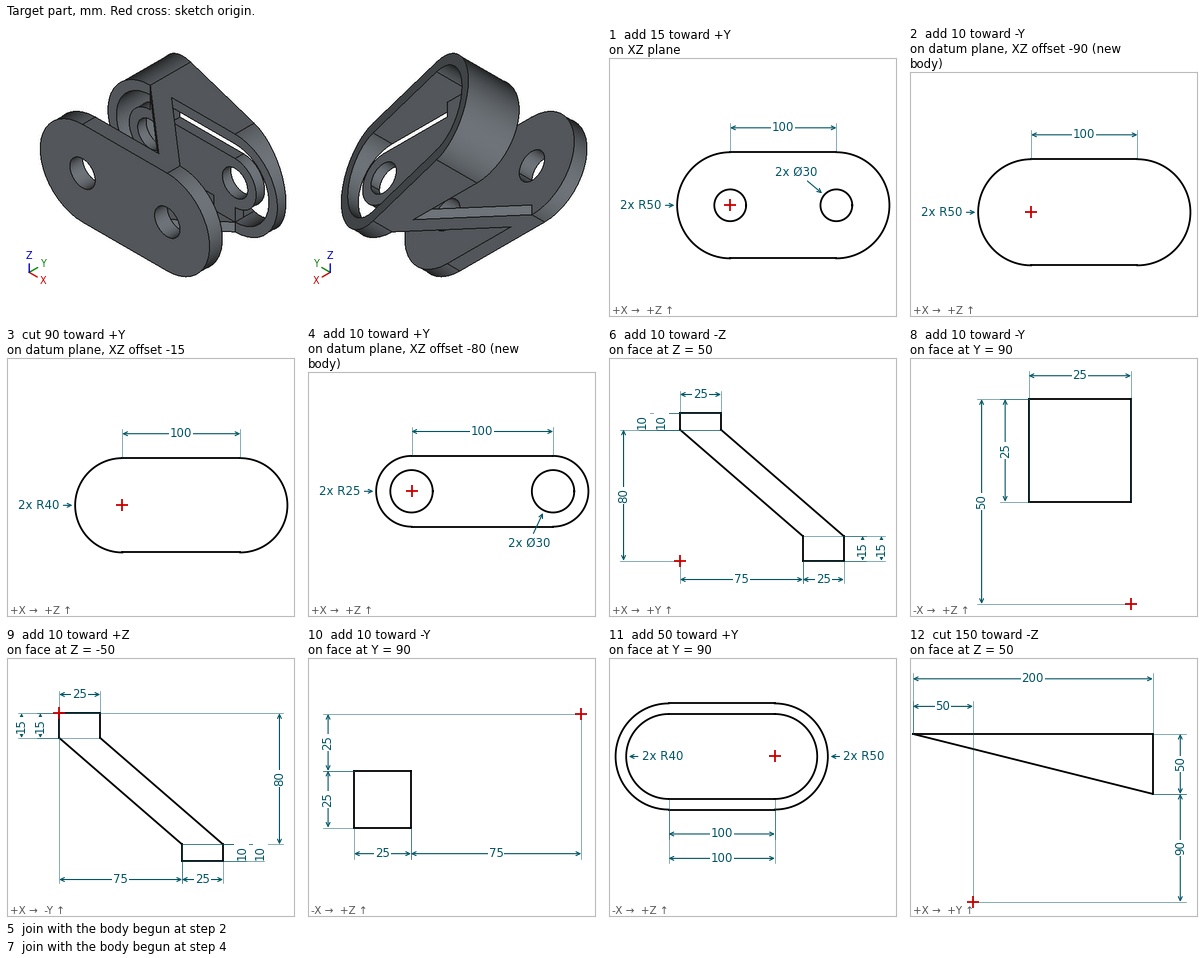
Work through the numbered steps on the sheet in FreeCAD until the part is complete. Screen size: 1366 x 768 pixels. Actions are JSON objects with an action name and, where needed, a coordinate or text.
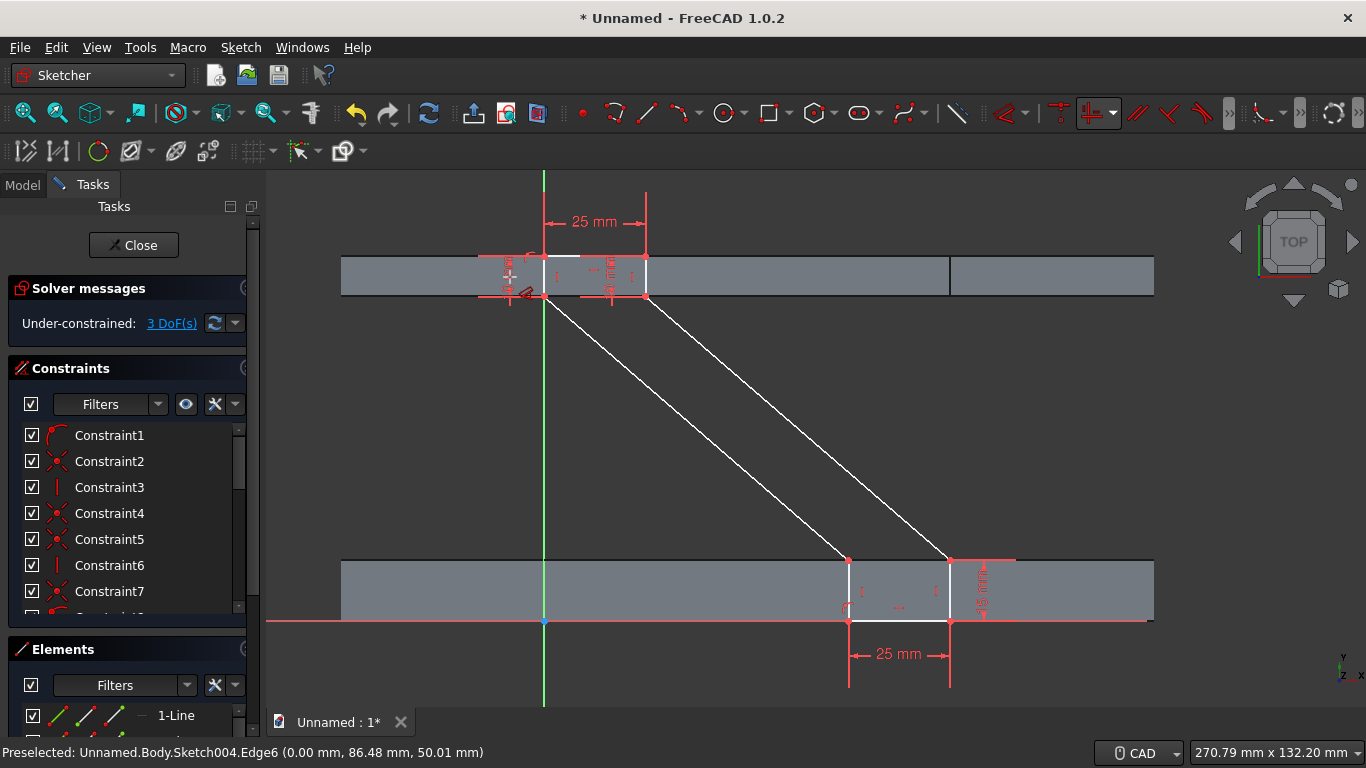
{"action": "left_click", "coordinate": [849, 579]}
{"action": "left_click", "coordinate": [883, 591]}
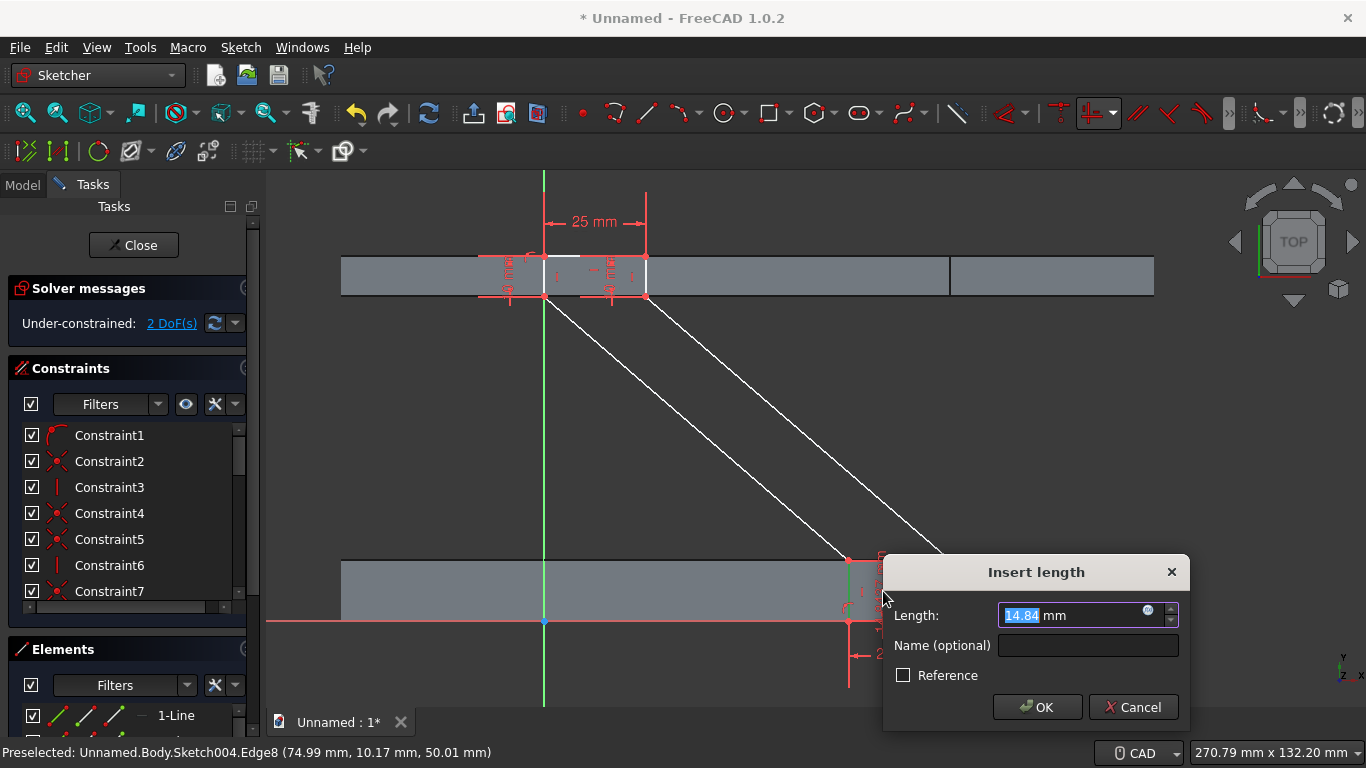
{"action": "type", "text": "15"}
{"action": "key", "text": "Return"}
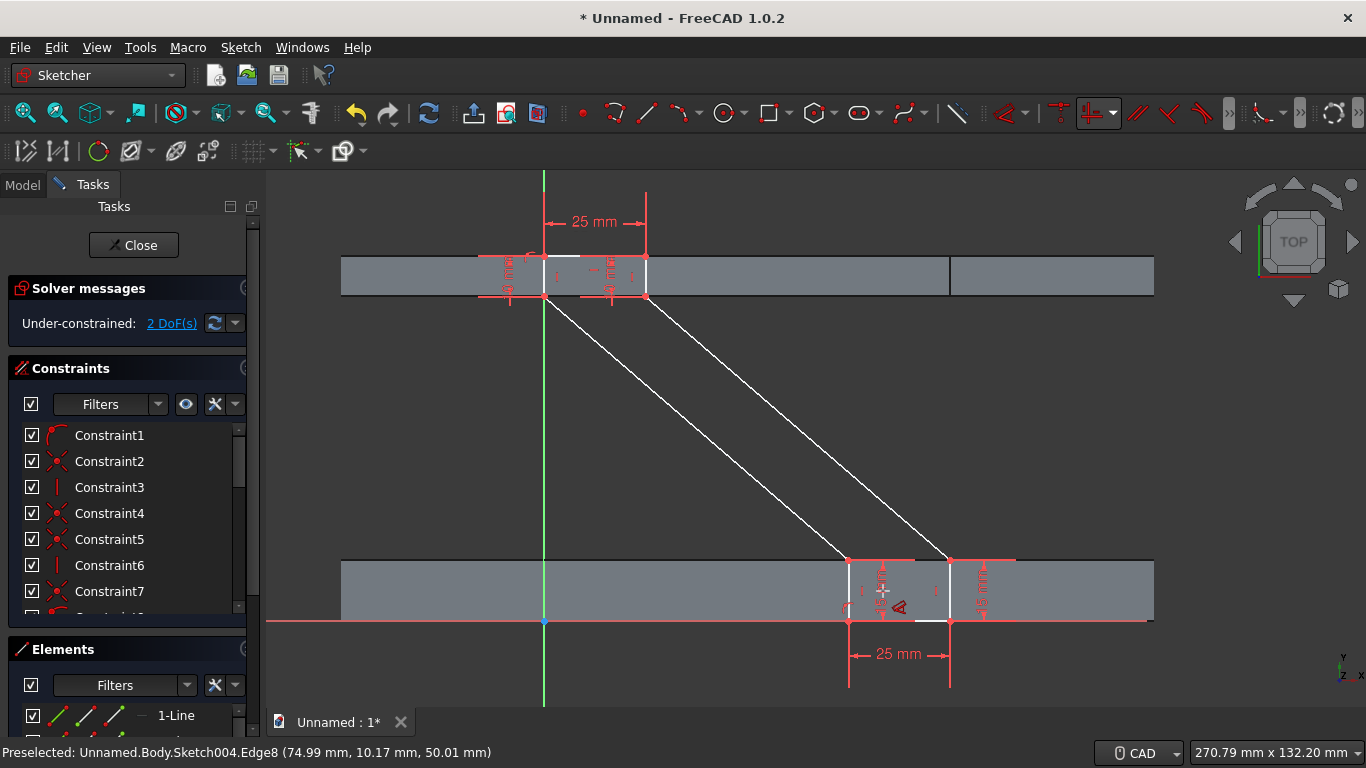
{"action": "left_click", "coordinate": [849, 621]}
{"action": "left_click", "coordinate": [696, 655]}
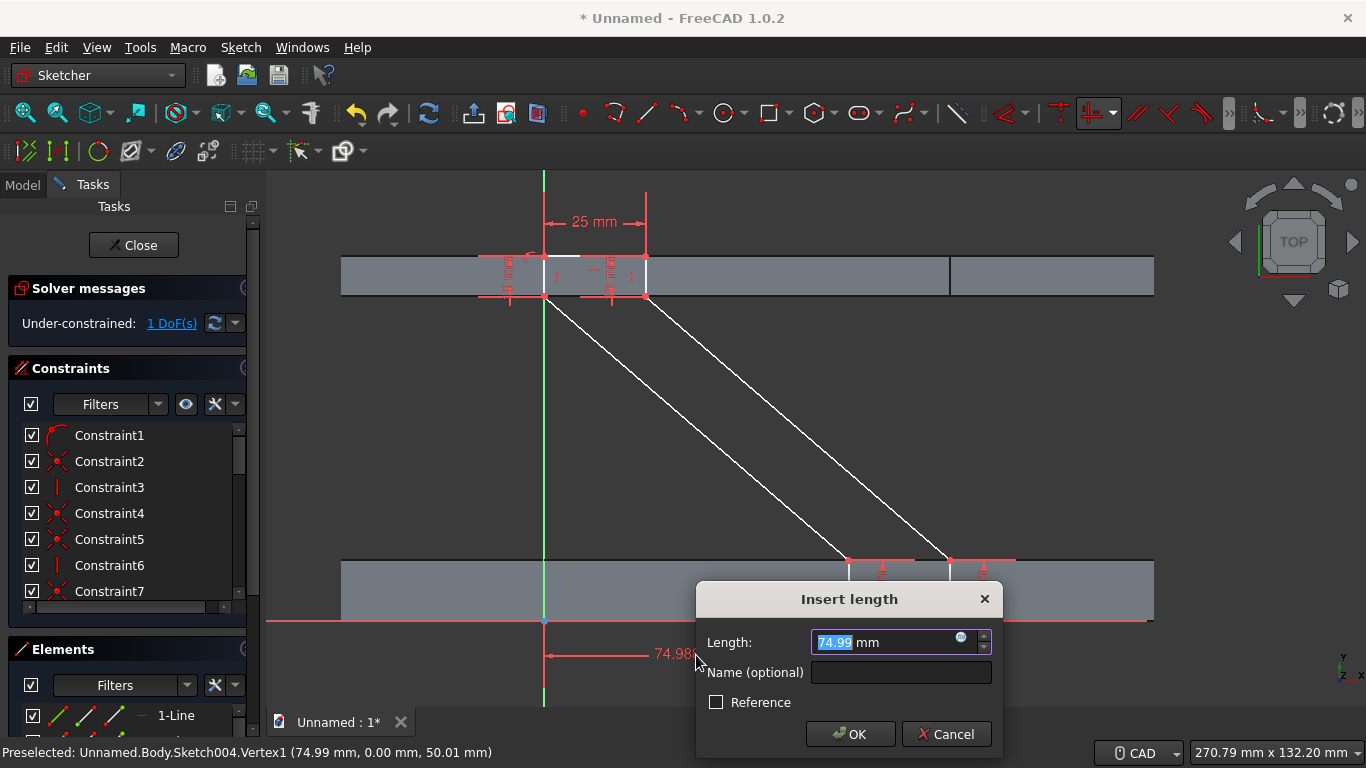
{"action": "type", "text": "75"}
{"action": "key", "text": "Return"}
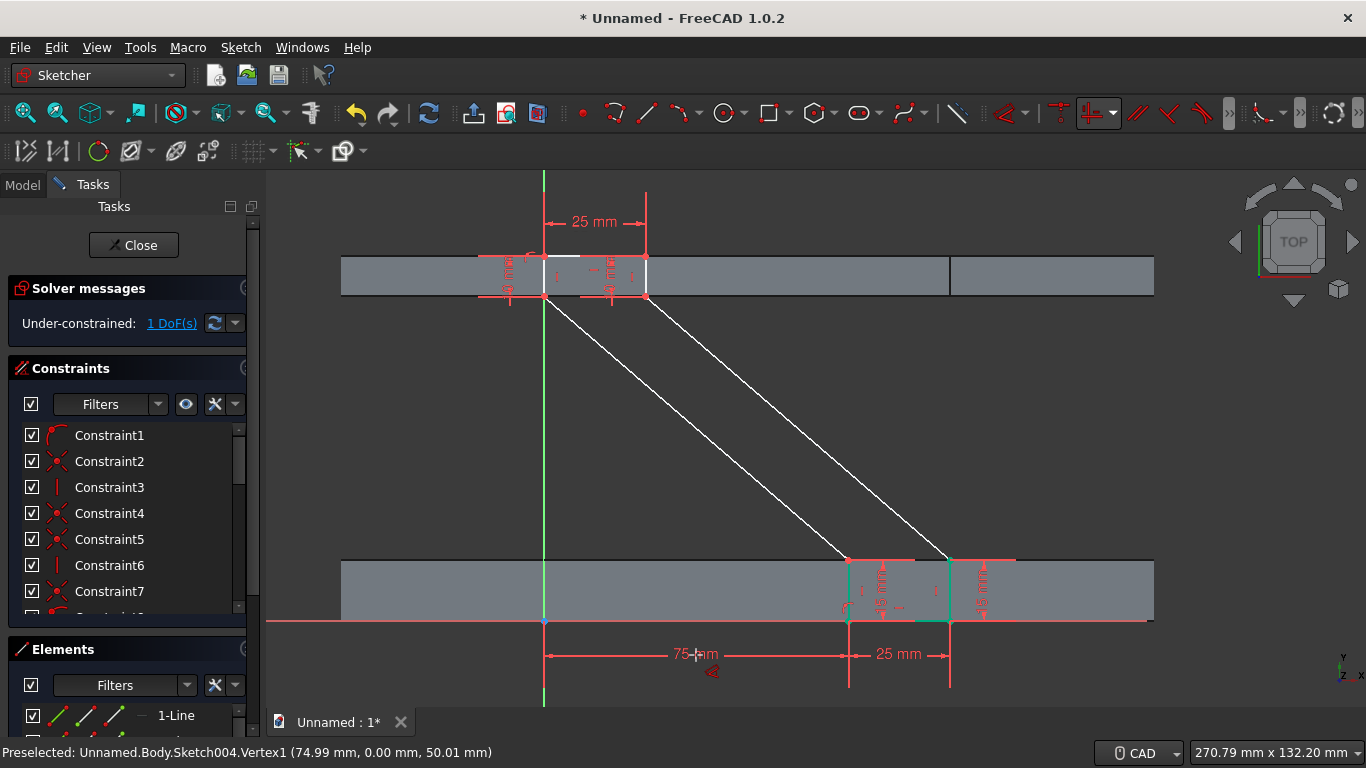
{"action": "left_click", "coordinate": [646, 297]}
{"action": "left_click", "coordinate": [510, 459]}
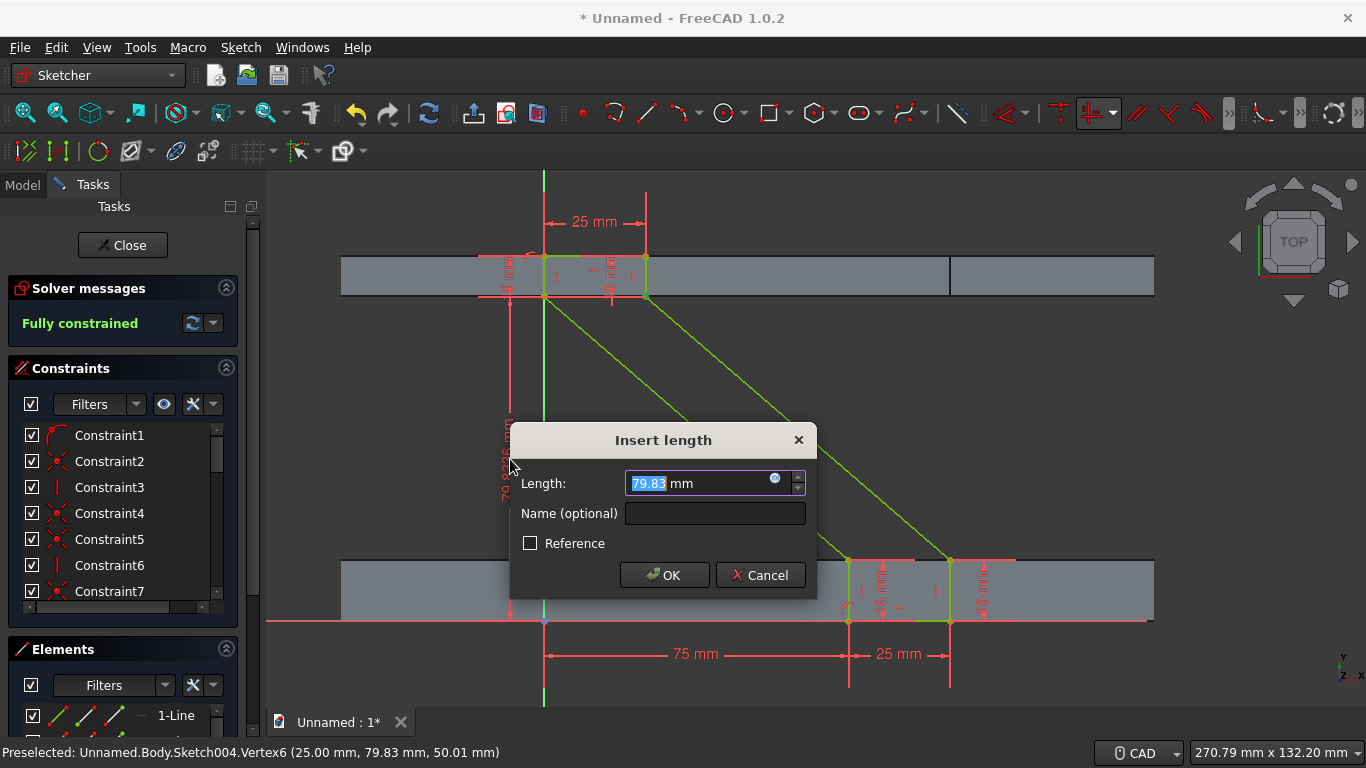
{"action": "type", "text": "80"}
{"action": "key", "text": "Return"}
{"action": "key", "text": "Escape"}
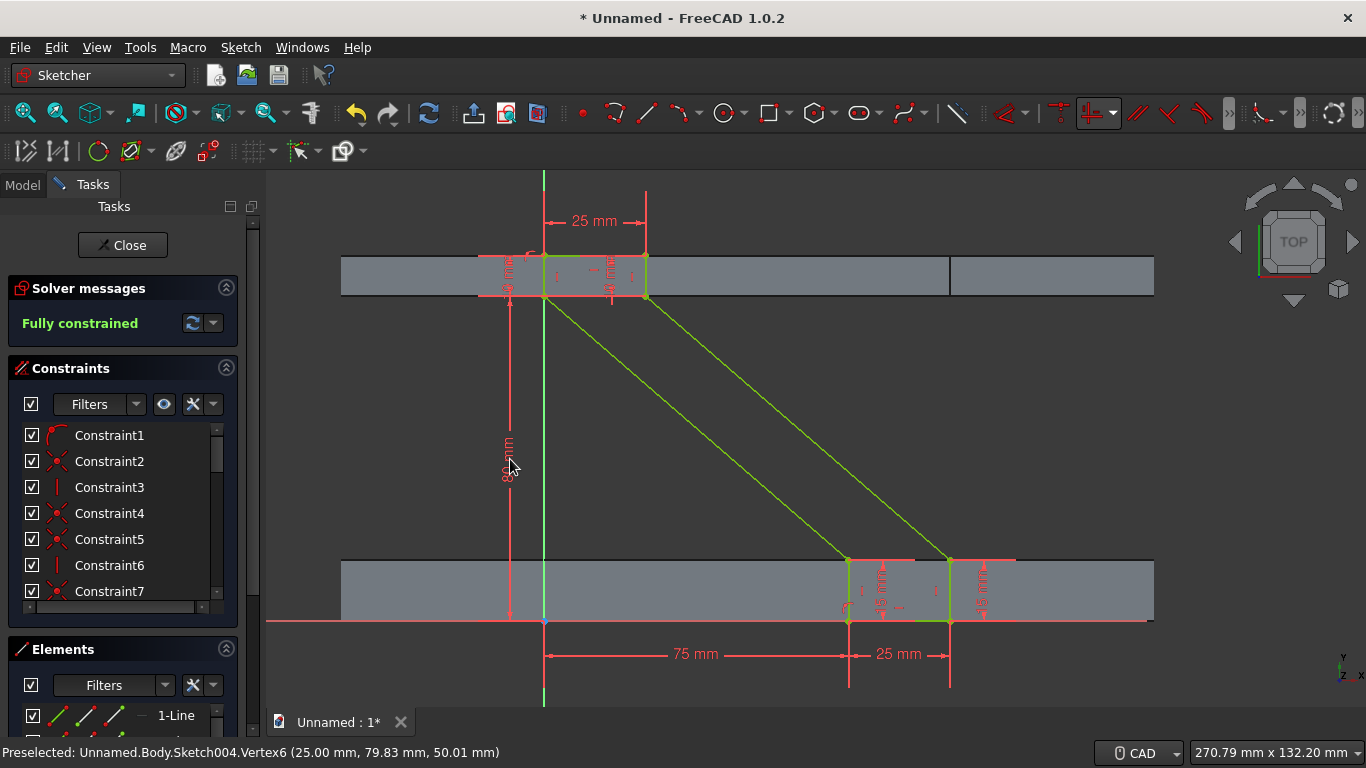
{"action": "left_click", "coordinate": [123, 245]}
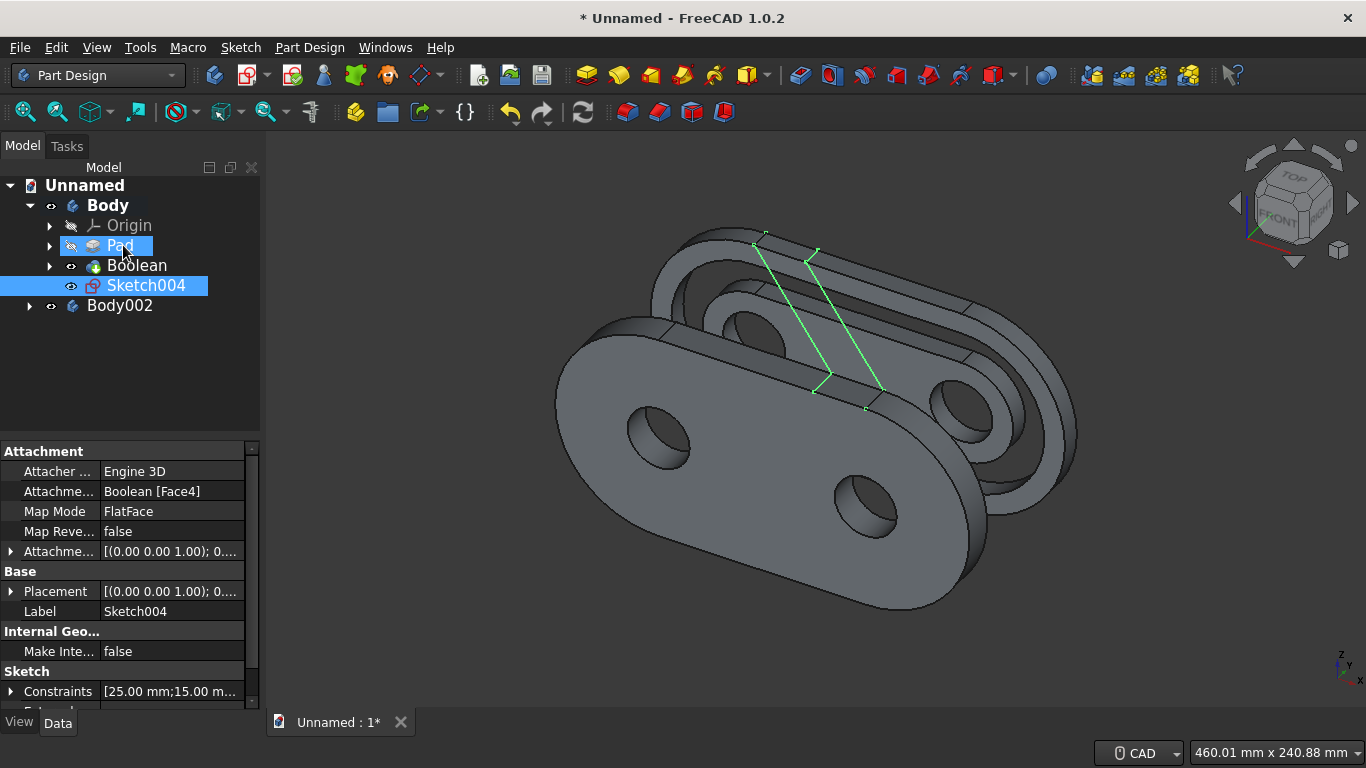
{"action": "left_click", "coordinate": [588, 76]}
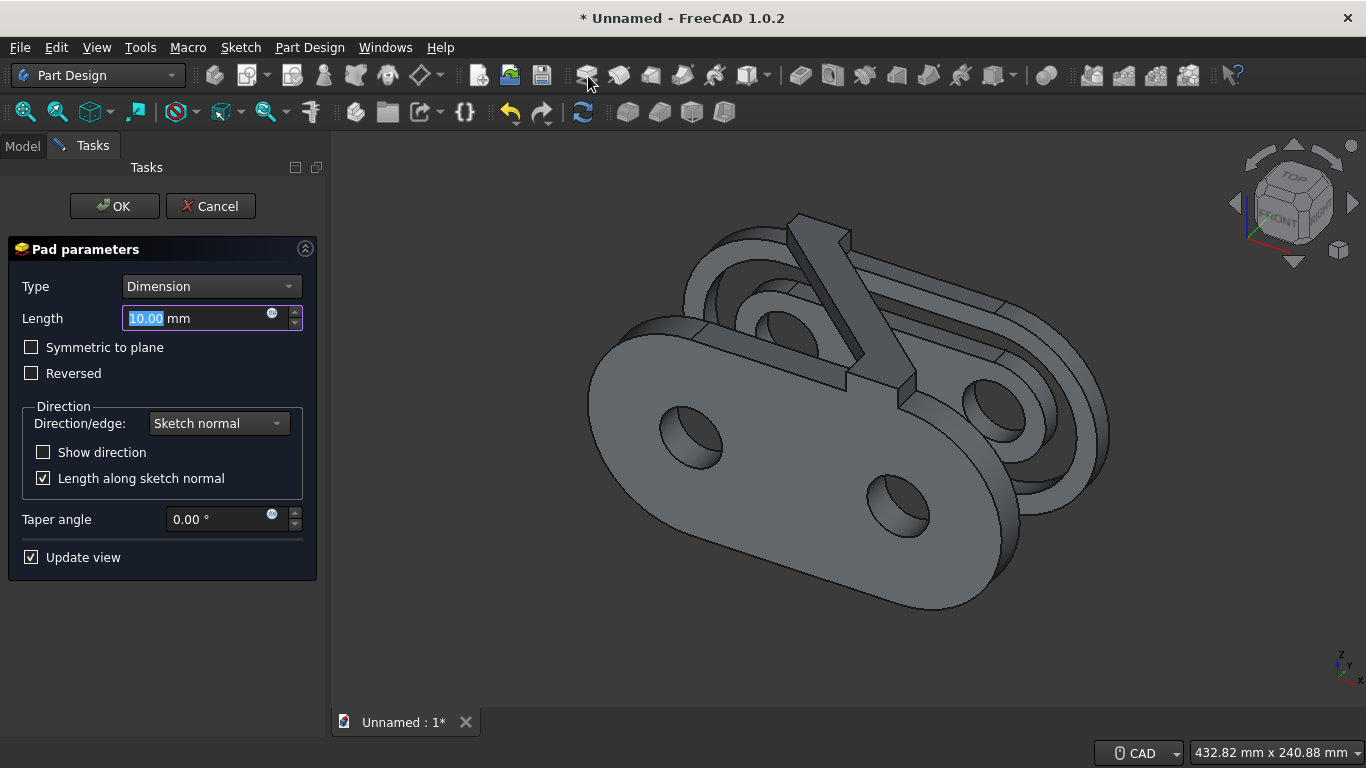
{"action": "type", "text": "10"}
{"action": "key", "text": "Tab"}